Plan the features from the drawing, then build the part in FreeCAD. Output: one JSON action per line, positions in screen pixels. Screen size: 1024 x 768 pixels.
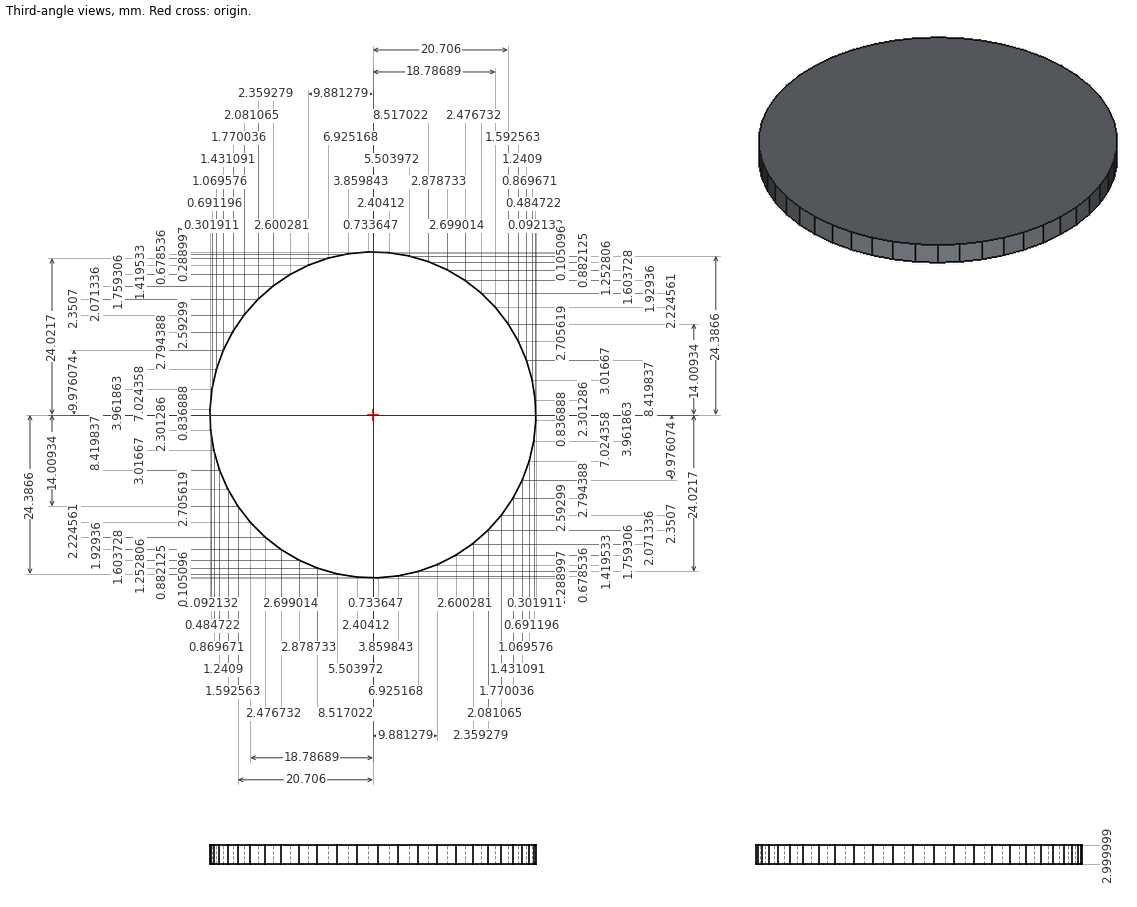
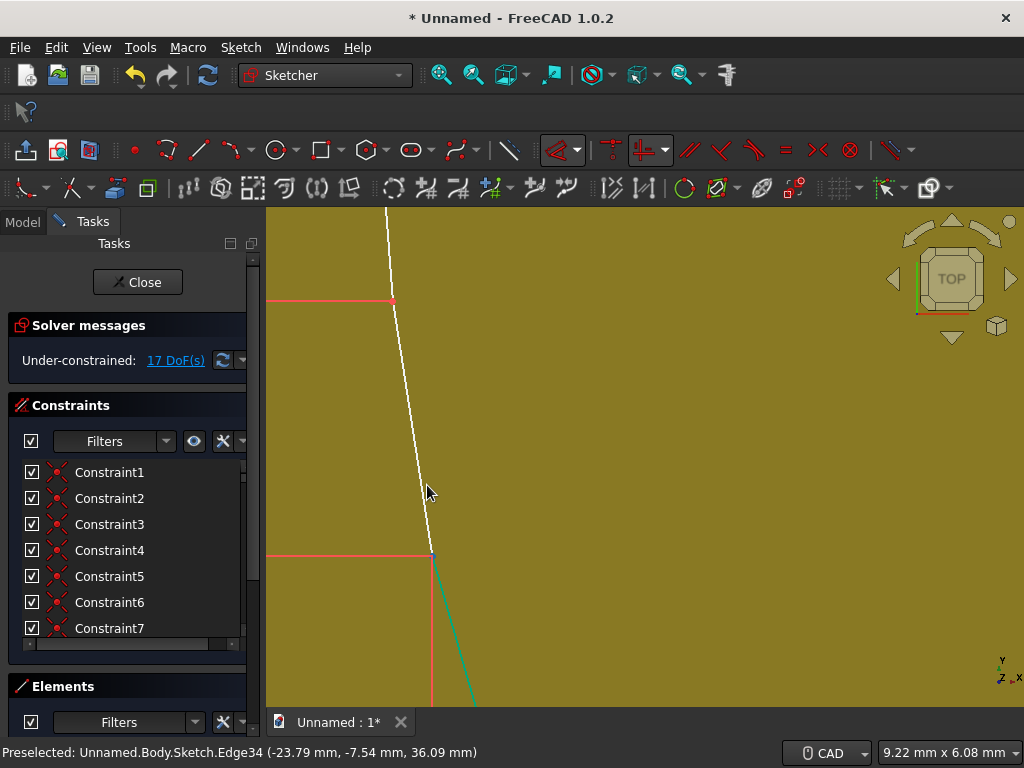
{"action": "left_click", "coordinate": [421, 480]}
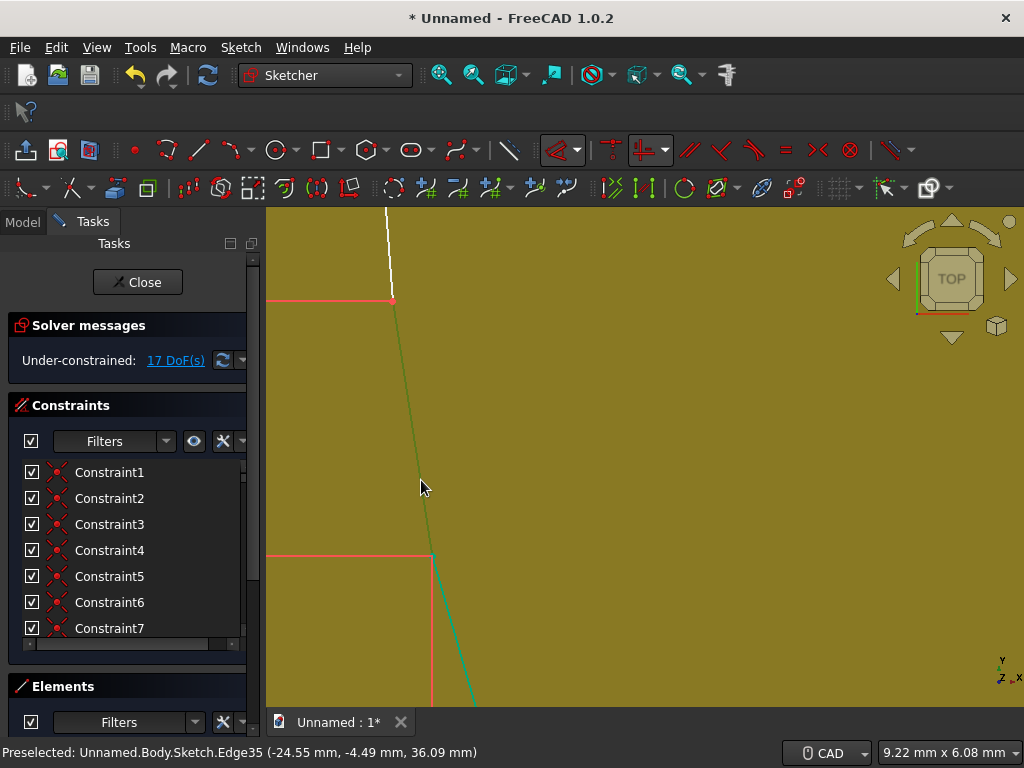
{"action": "key", "text": "l"}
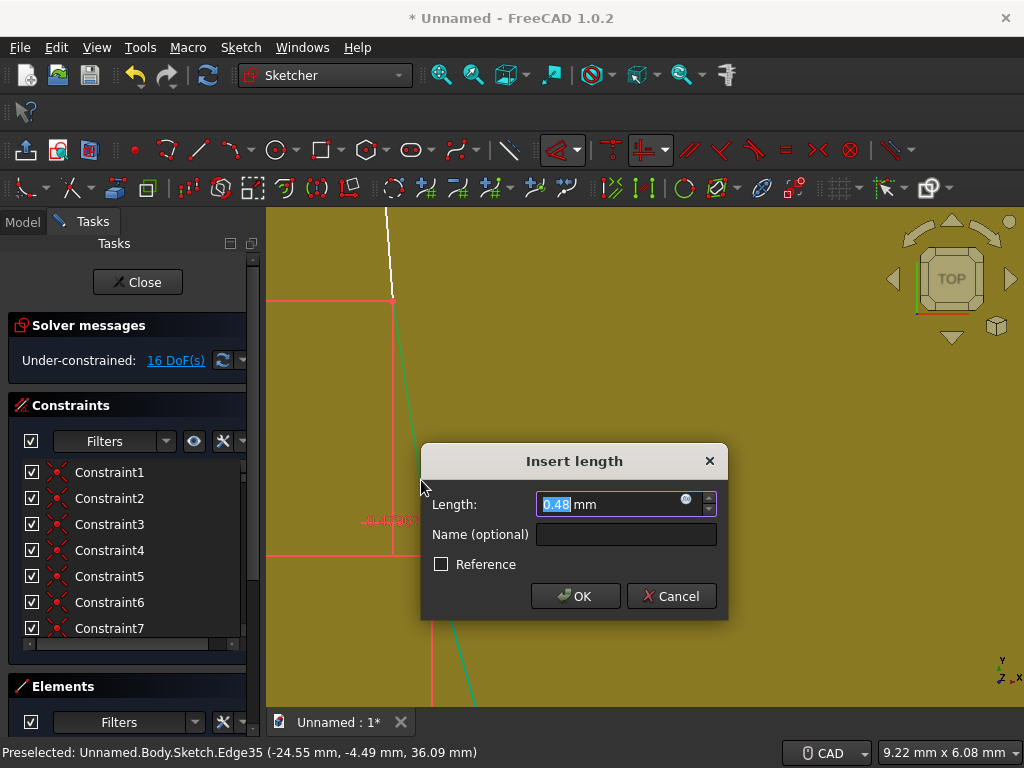
{"action": "type", "text": "0.484722"}
{"action": "key", "text": "Return"}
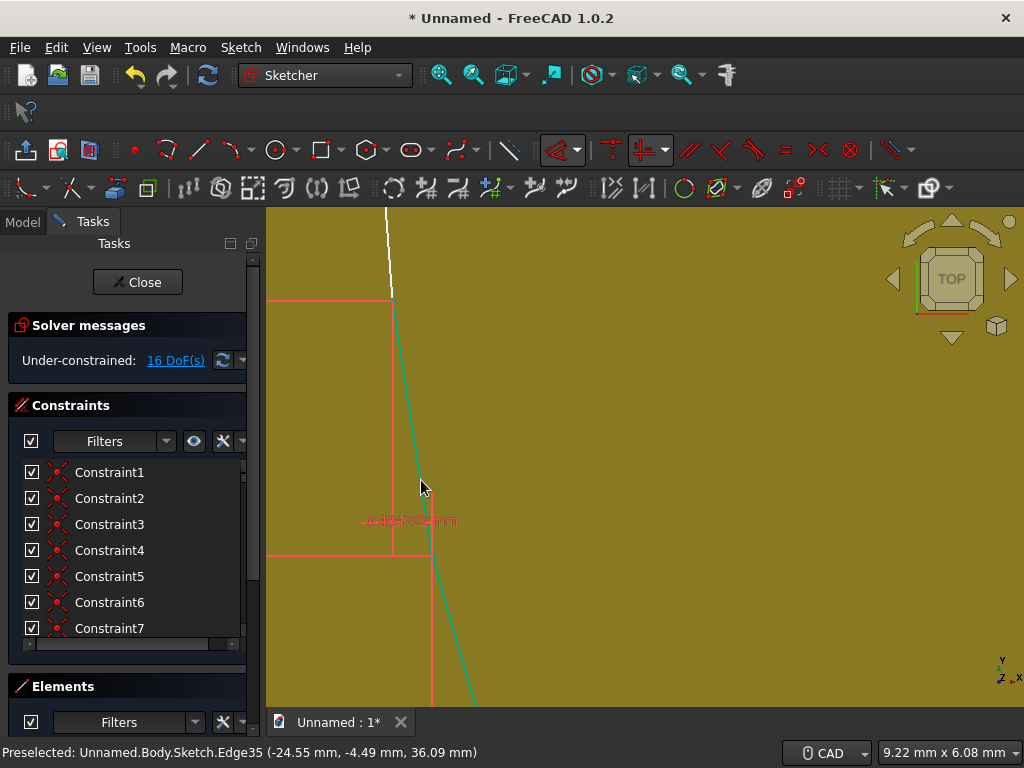
{"action": "scroll", "coordinate": [389, 250], "scroll_direction": "up", "scroll_amount": 9}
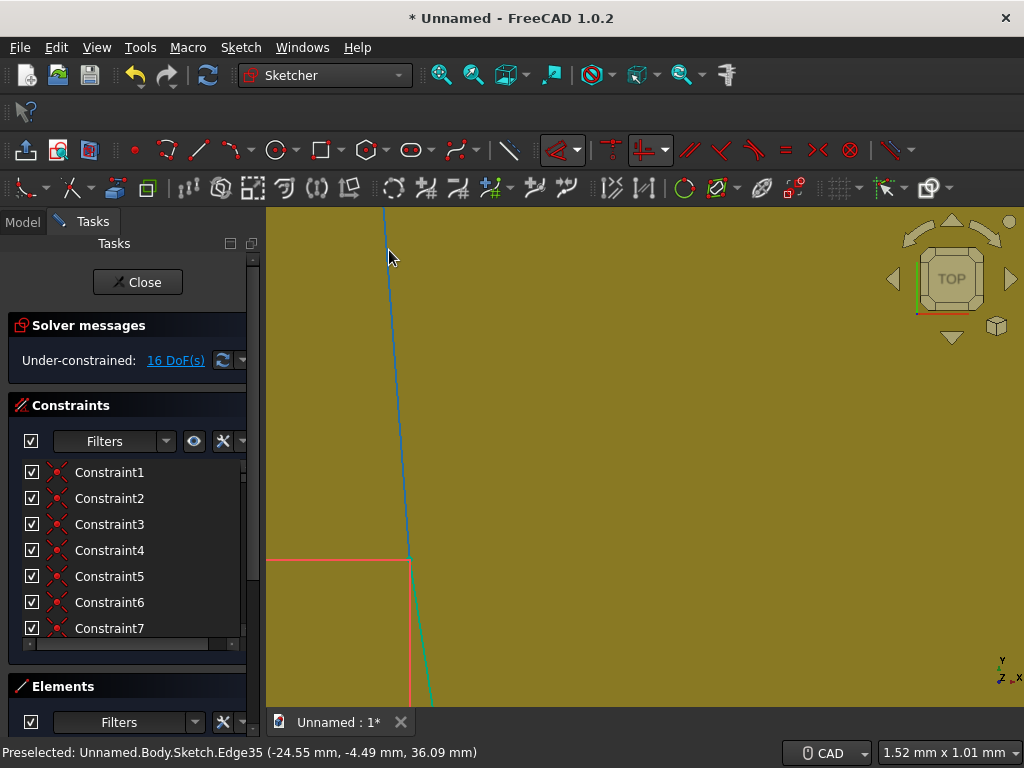
{"action": "left_click", "coordinate": [386, 248]}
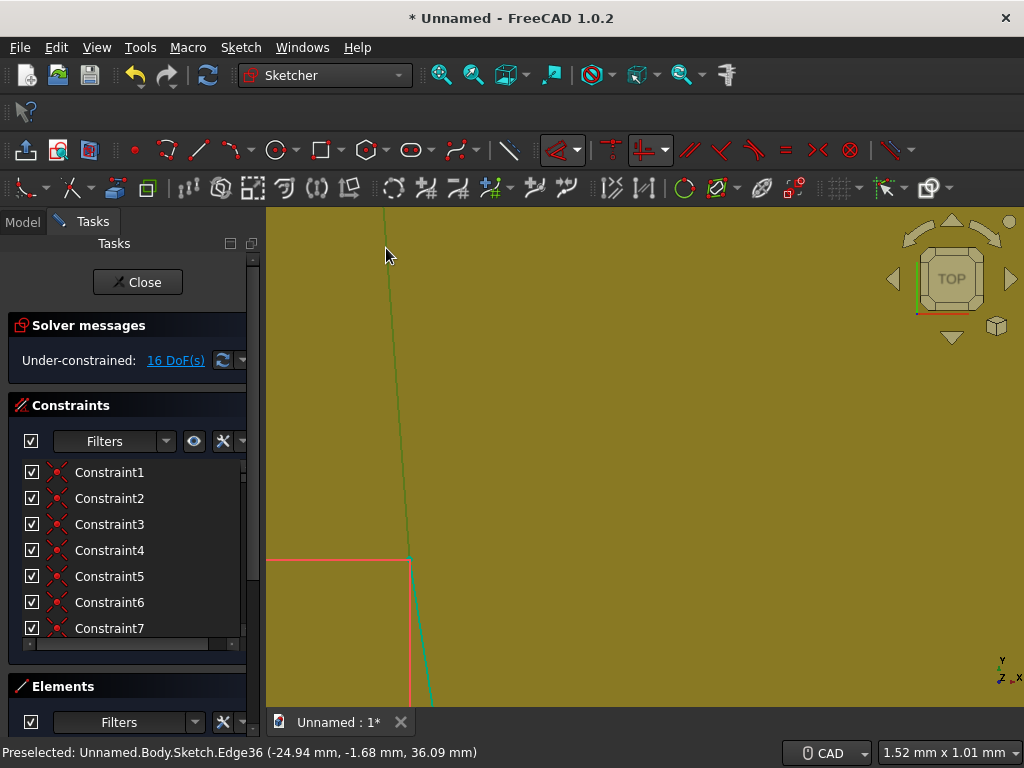
{"action": "left_click", "coordinate": [580, 150]}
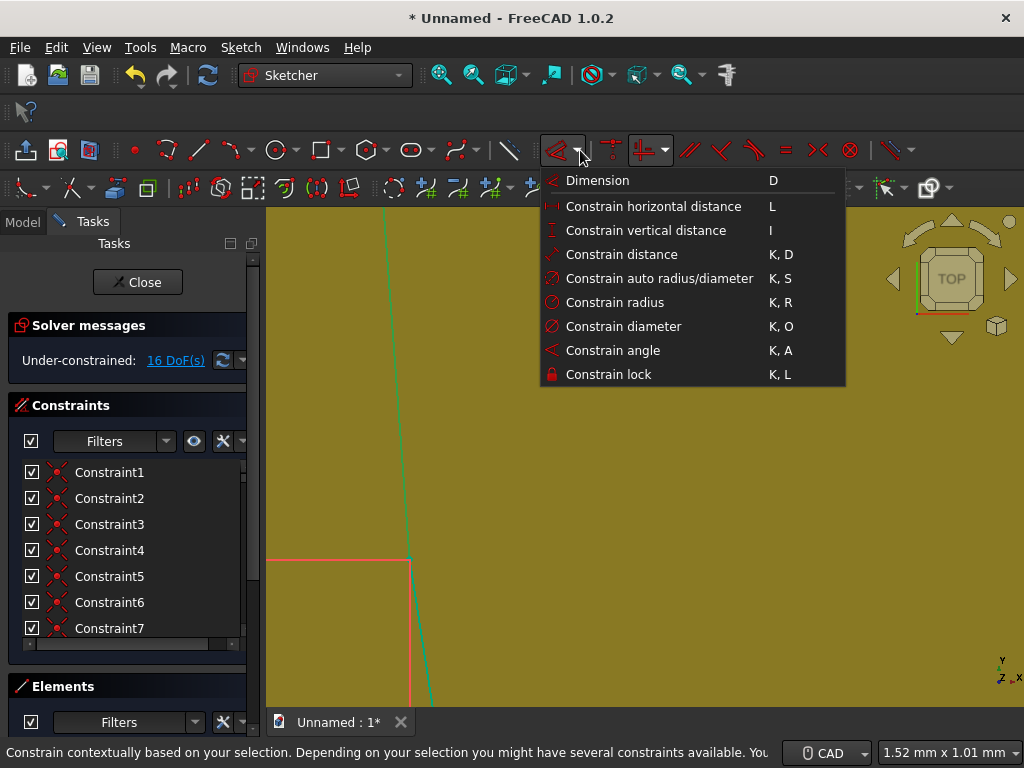
{"action": "left_click", "coordinate": [693, 206]}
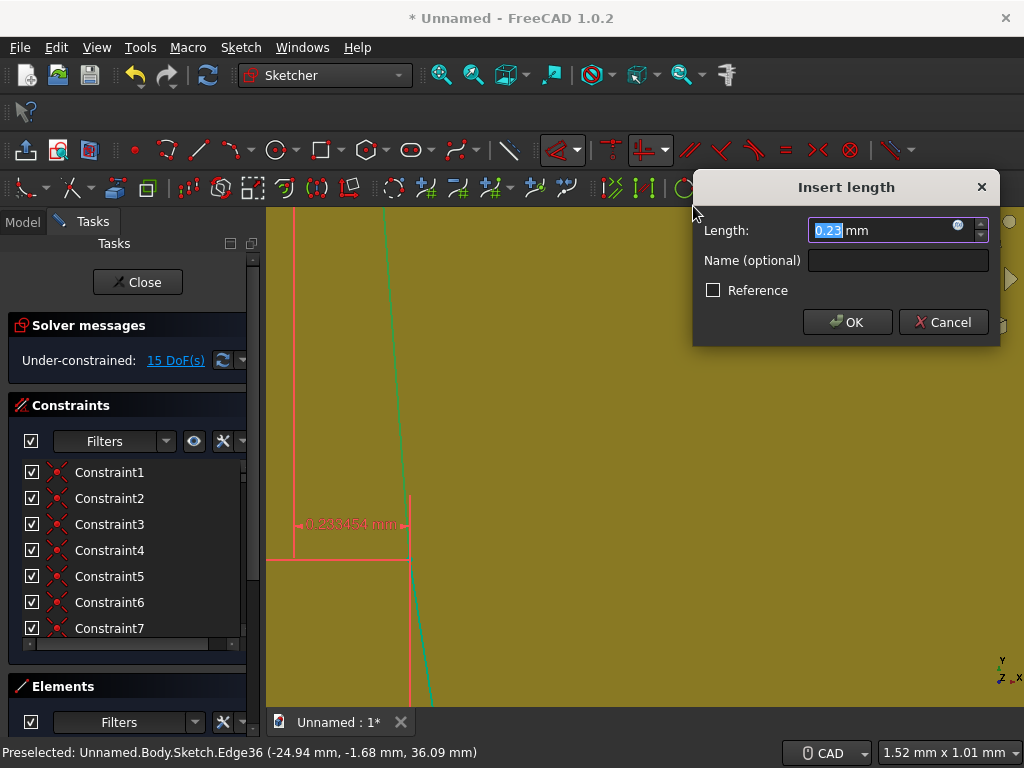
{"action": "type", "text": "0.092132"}
{"action": "key", "text": "Return"}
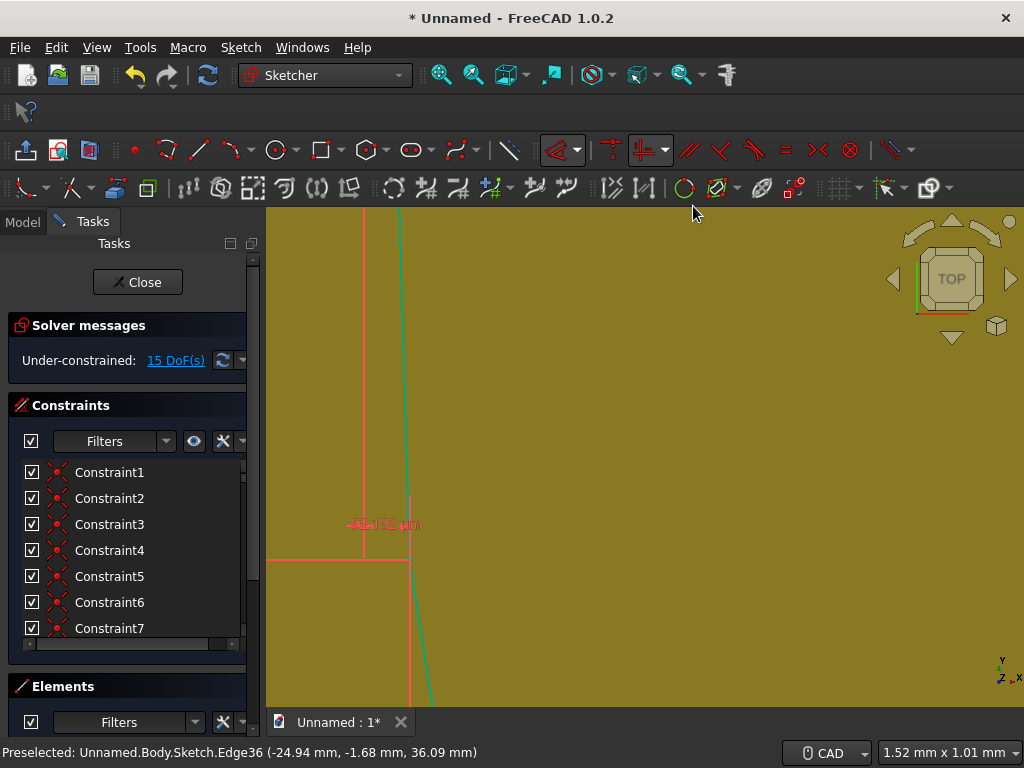
{"action": "scroll", "coordinate": [576, 457], "scroll_direction": "down", "scroll_amount": 15}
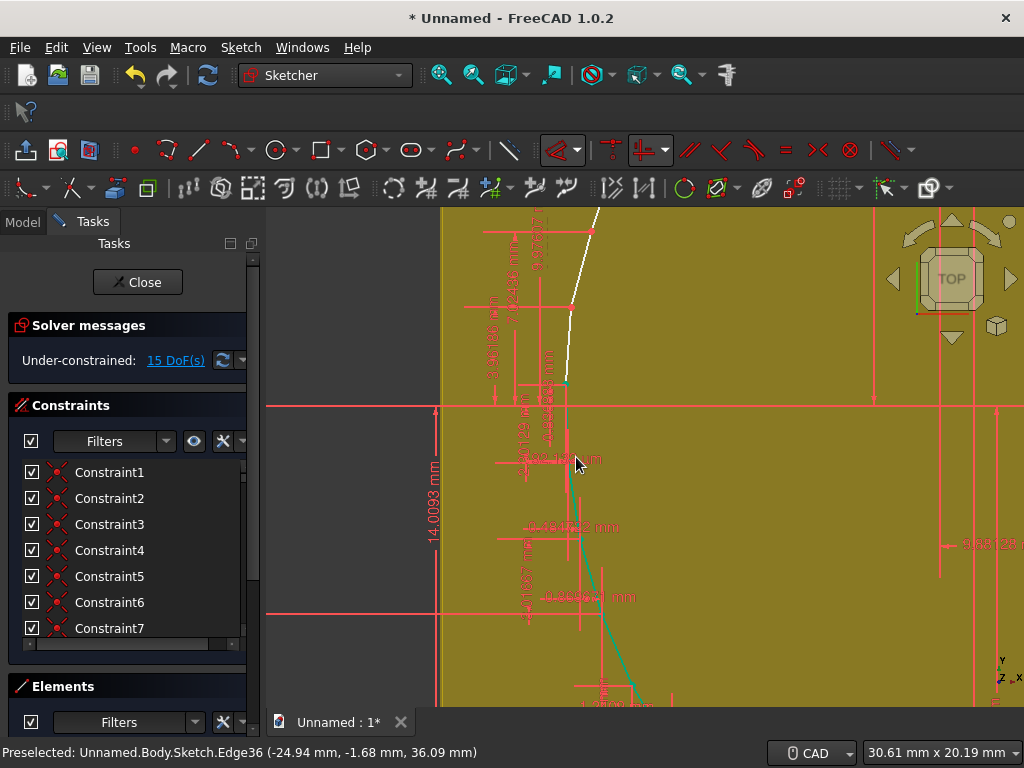
{"action": "scroll", "coordinate": [377, 474], "scroll_direction": "down", "scroll_amount": 7}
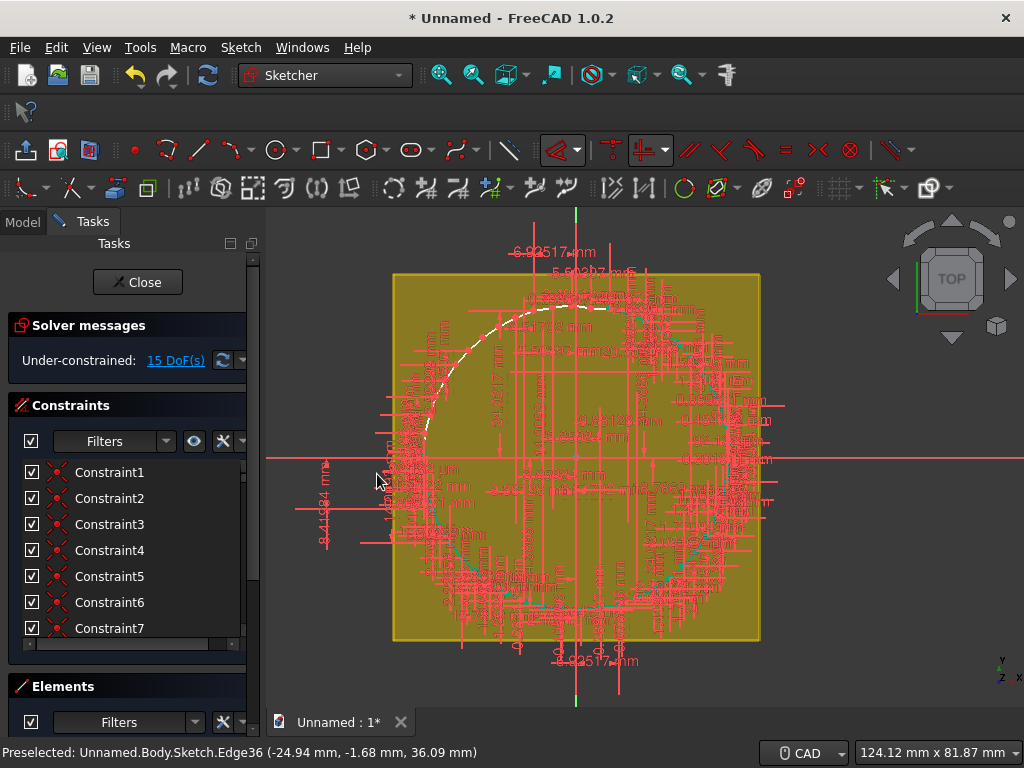
{"action": "scroll", "coordinate": [424, 447], "scroll_direction": "up", "scroll_amount": 16}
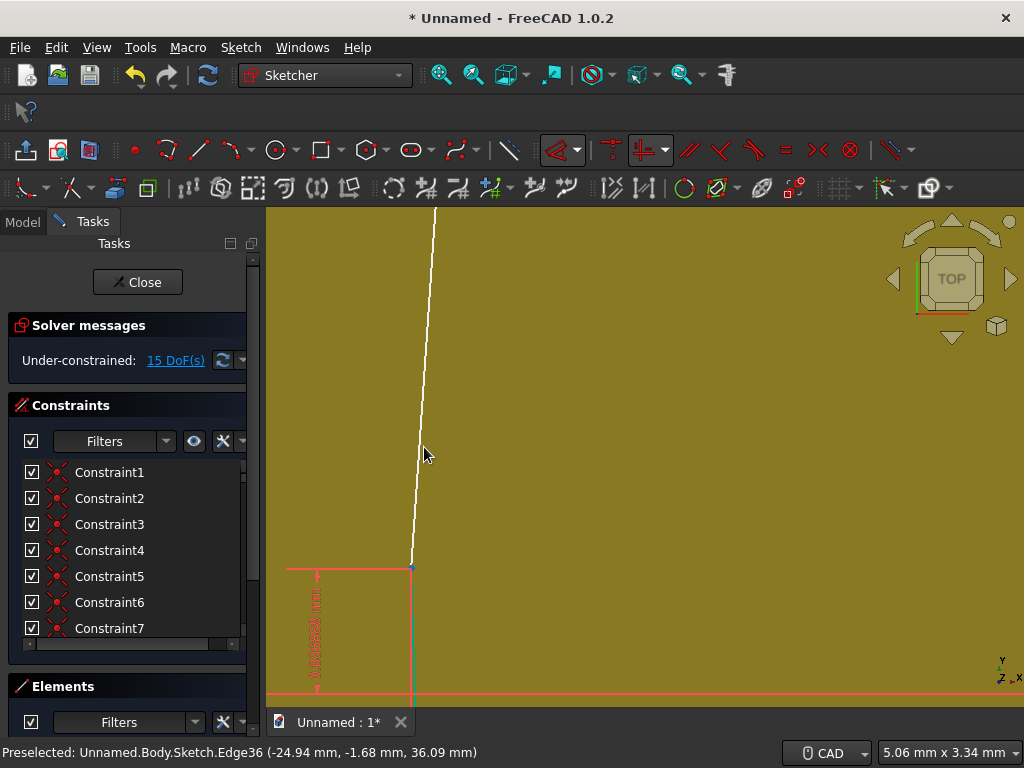
{"action": "left_click", "coordinate": [421, 428]}